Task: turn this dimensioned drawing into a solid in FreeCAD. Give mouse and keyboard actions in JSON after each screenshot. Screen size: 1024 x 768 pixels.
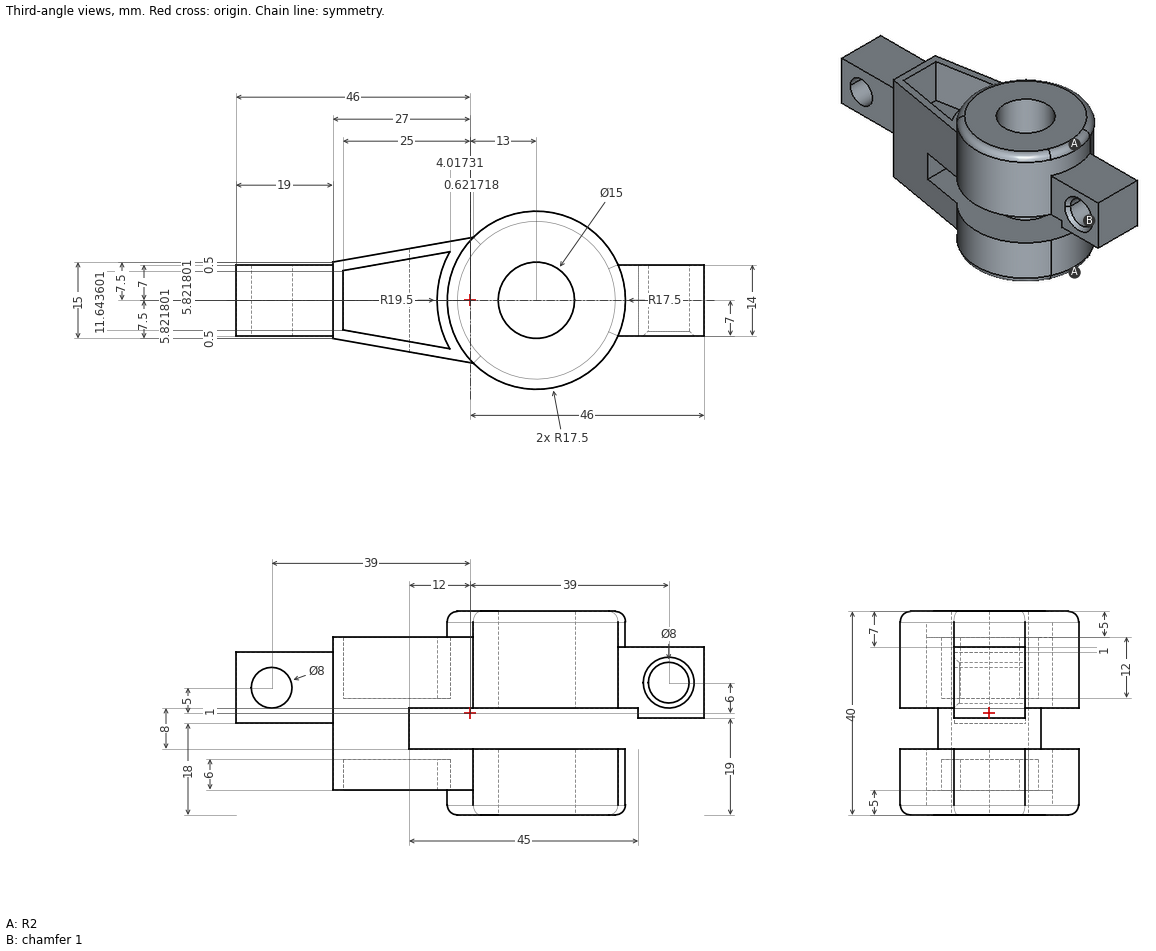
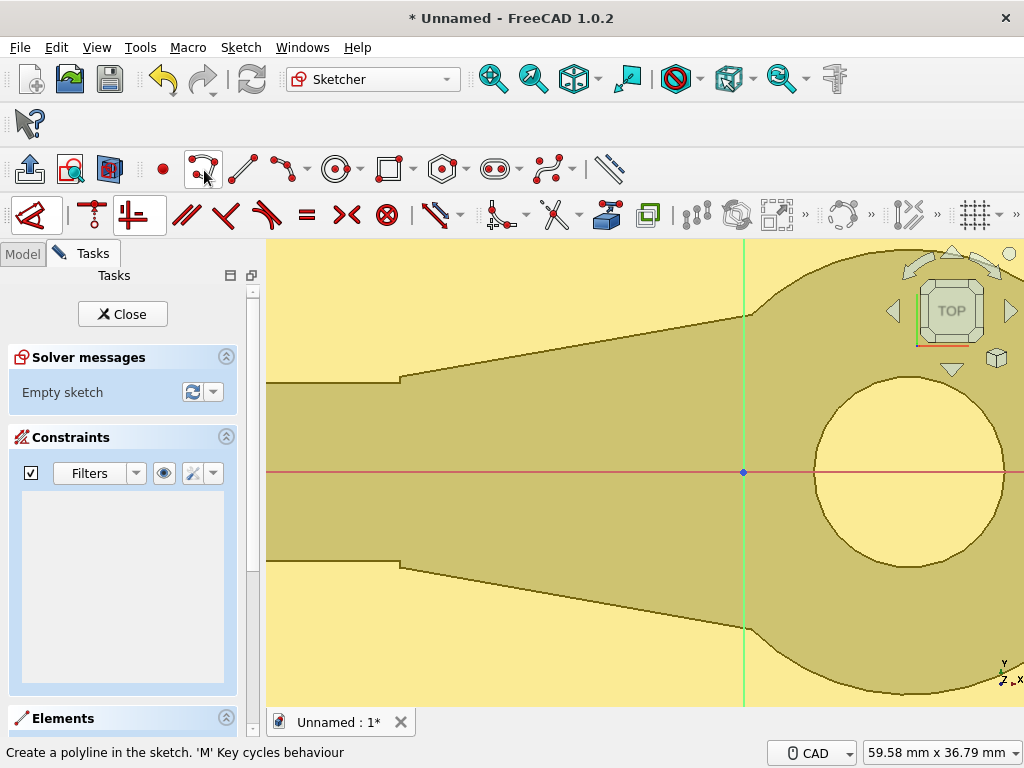
{"action": "scroll", "coordinate": [752, 630], "scroll_direction": "up", "scroll_amount": 4}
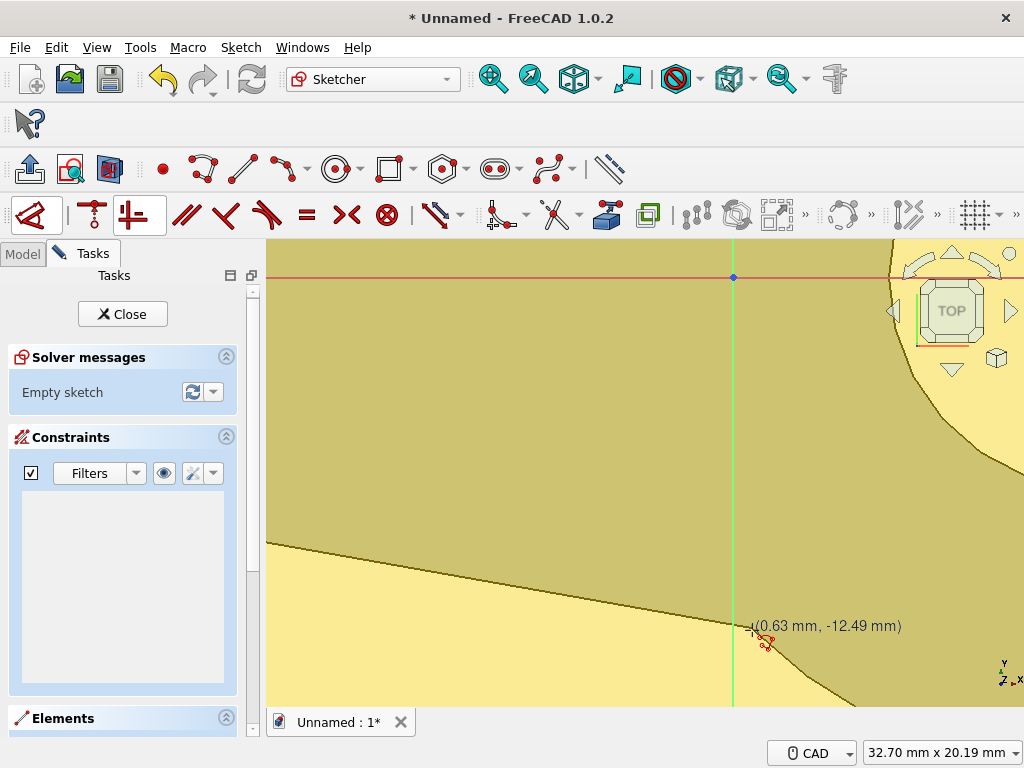
{"action": "left_click", "coordinate": [751, 628]}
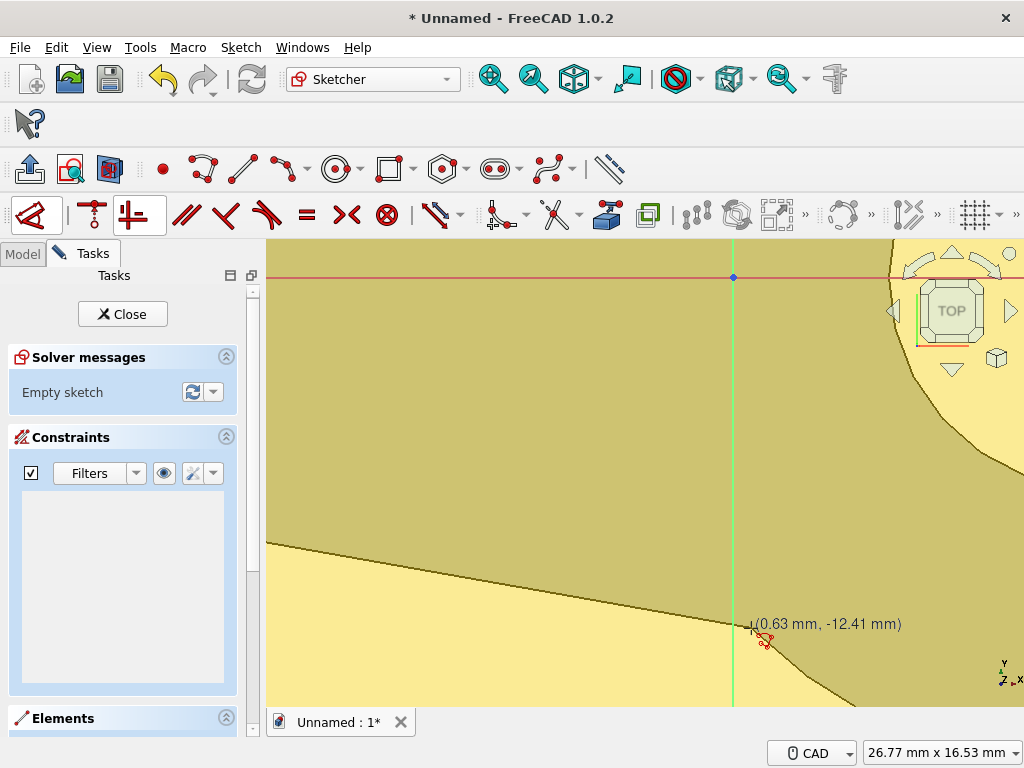
{"action": "scroll", "coordinate": [753, 632], "scroll_direction": "down", "scroll_amount": 4}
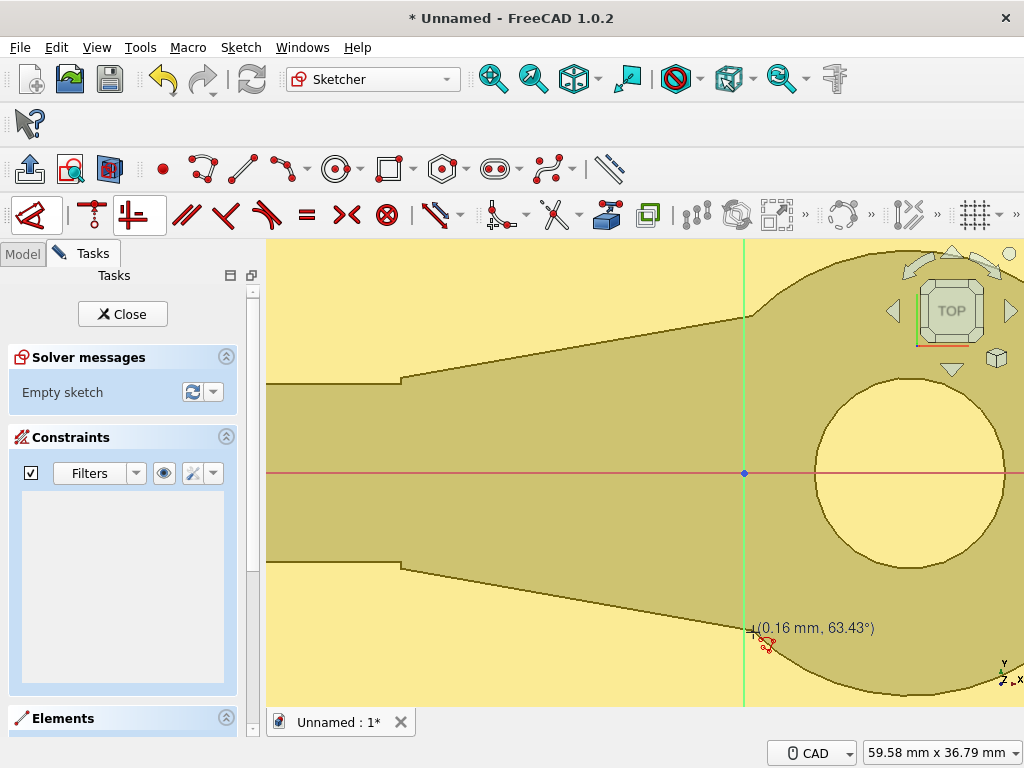
{"action": "left_click", "coordinate": [401, 569]}
{"action": "left_click", "coordinate": [401, 378]}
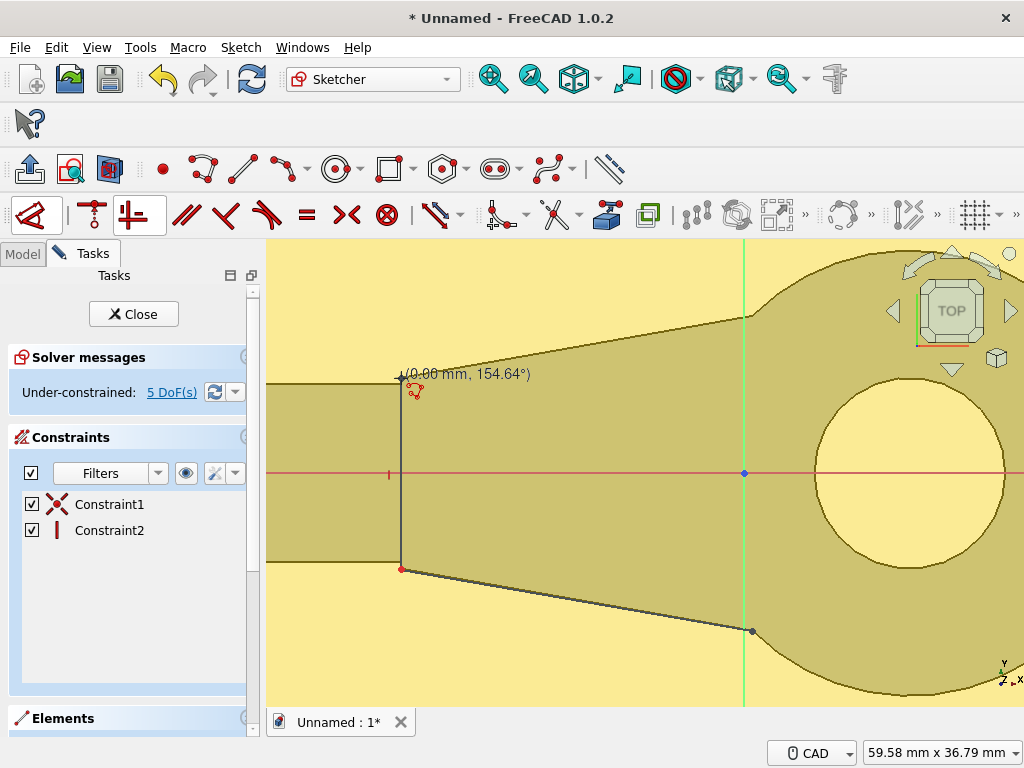
{"action": "scroll", "coordinate": [752, 316], "scroll_direction": "up", "scroll_amount": 4}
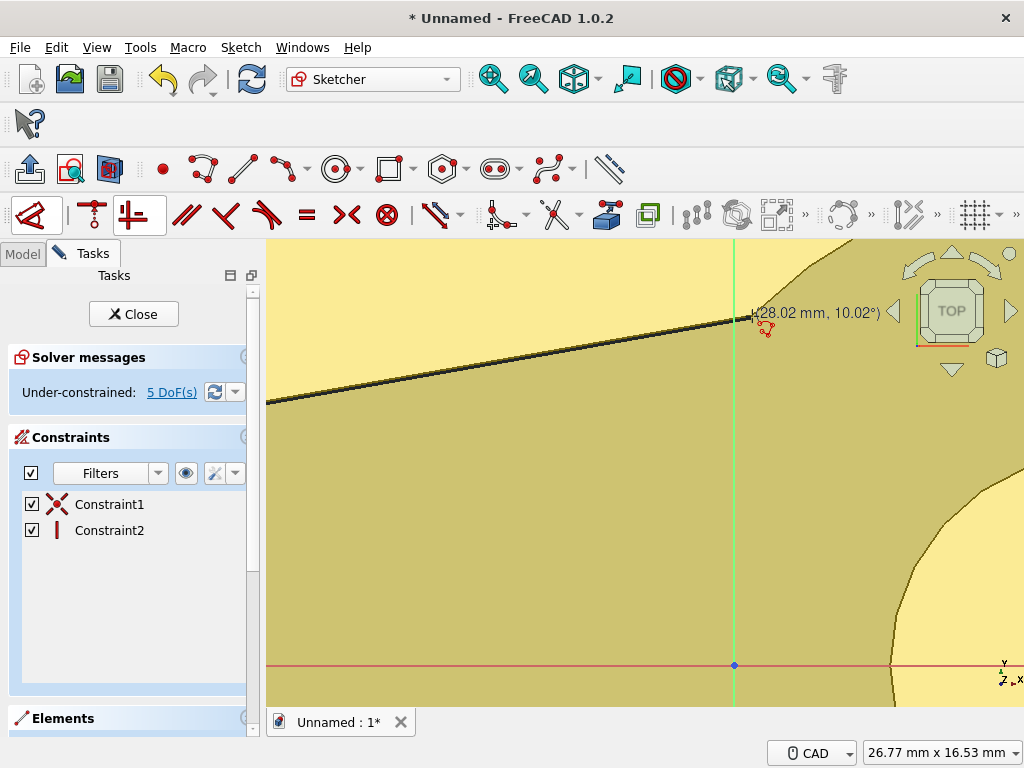
{"action": "left_click", "coordinate": [752, 316]}
{"action": "right_click", "coordinate": [752, 316]}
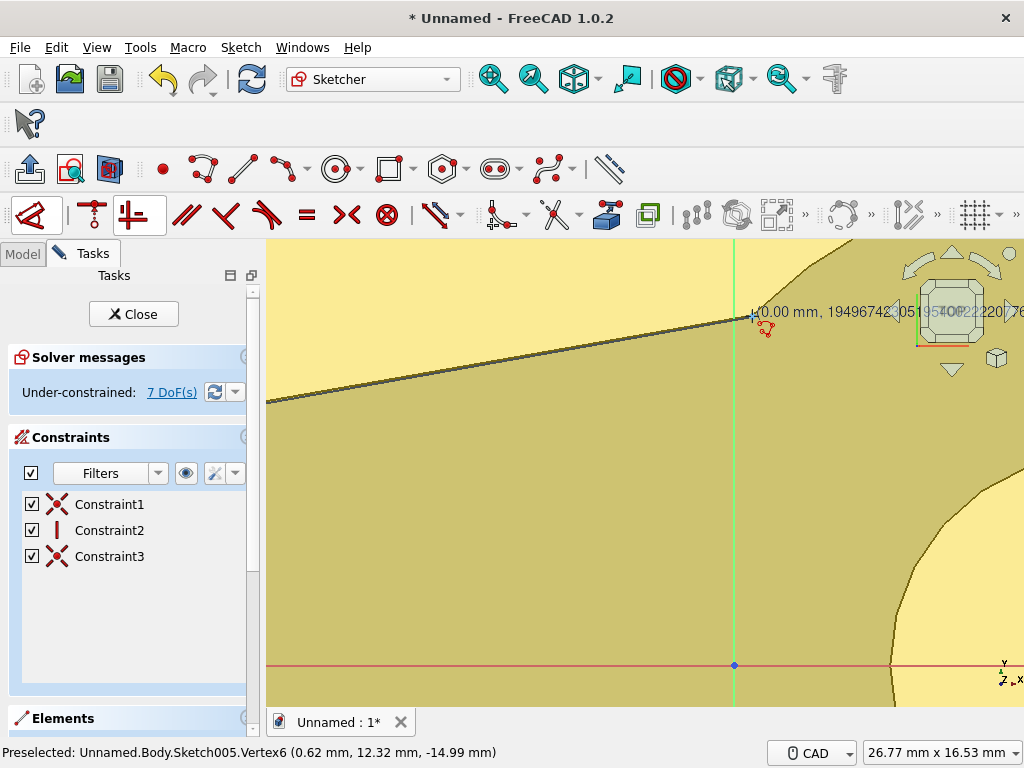
{"action": "left_click", "coordinate": [284, 170]}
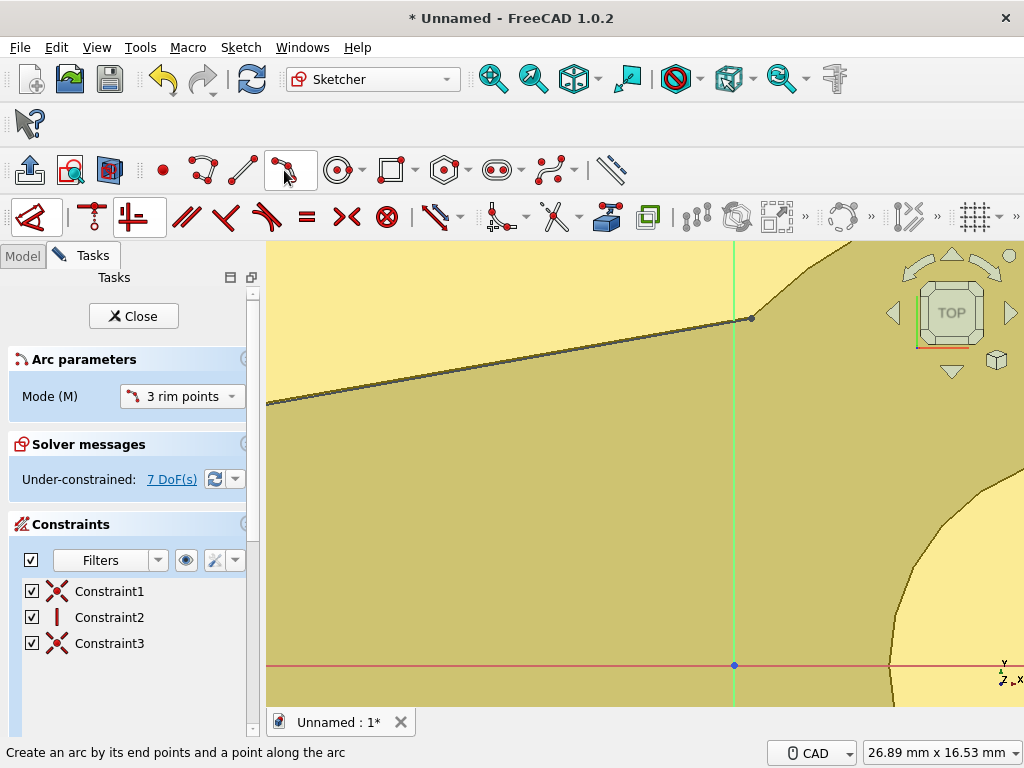
{"action": "left_click", "coordinate": [752, 319]}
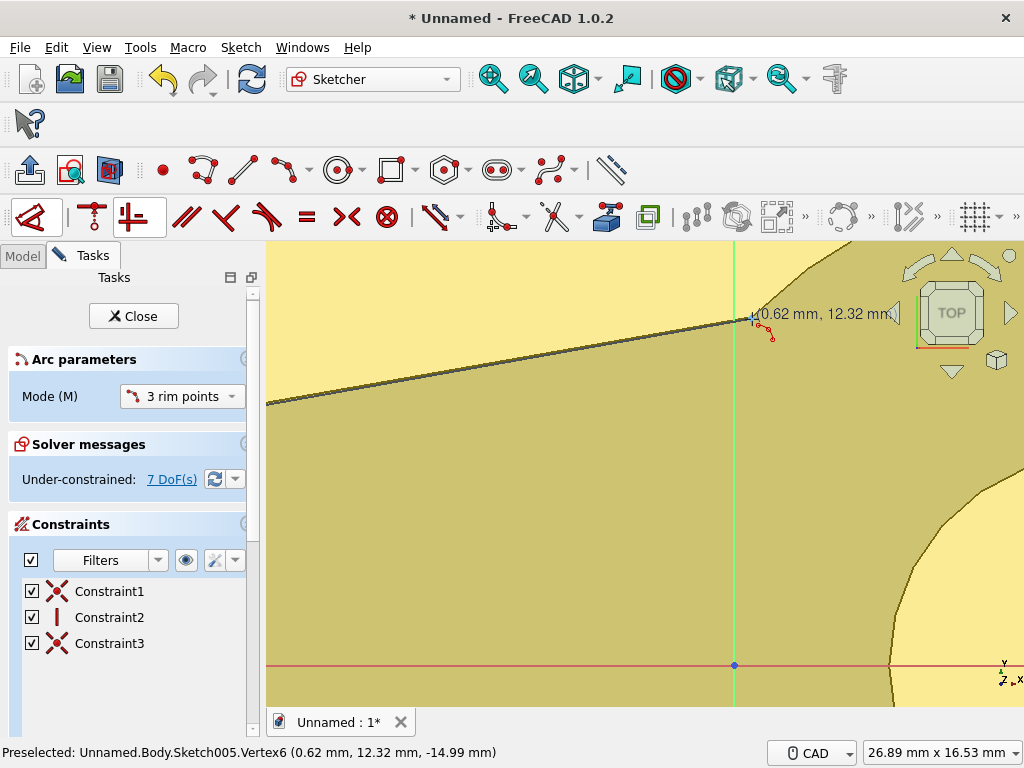
{"action": "scroll", "coordinate": [751, 317], "scroll_direction": "down", "scroll_amount": 4}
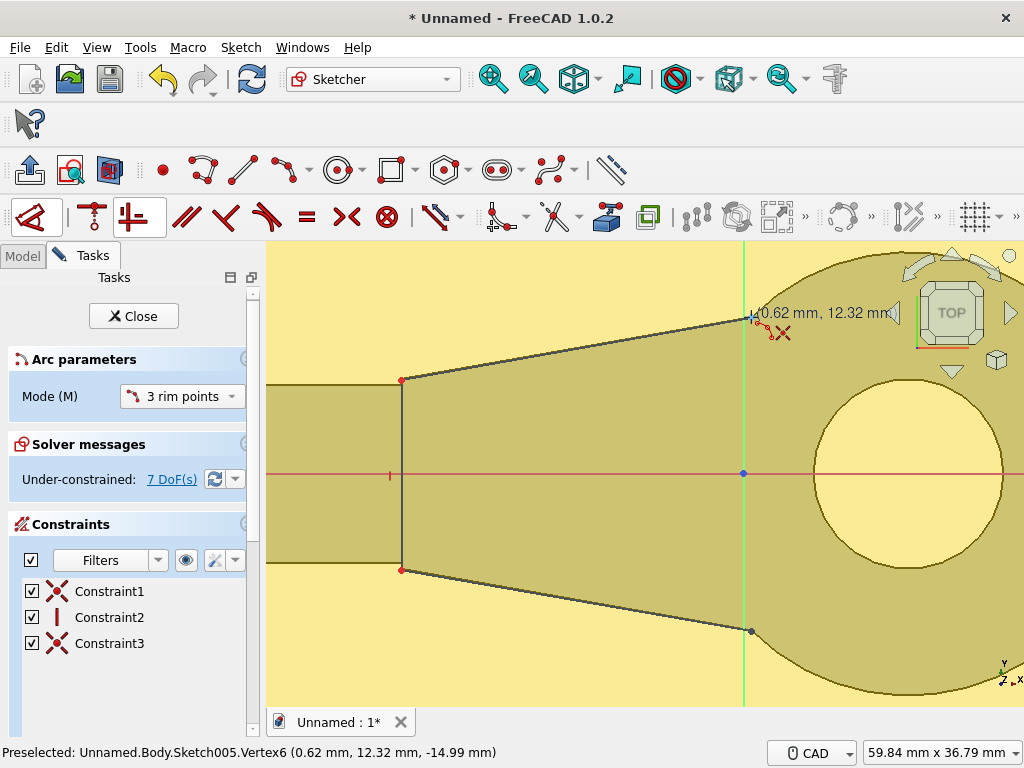
{"action": "scroll", "coordinate": [752, 631], "scroll_direction": "up", "scroll_amount": 4}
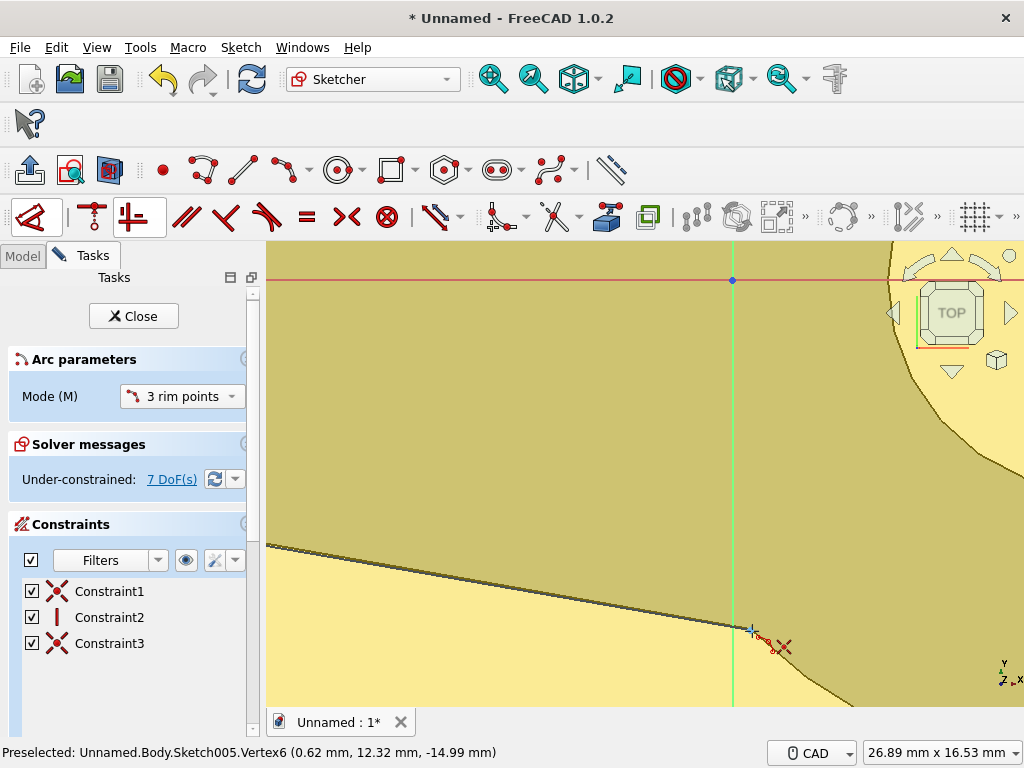
{"action": "left_click", "coordinate": [751, 630]}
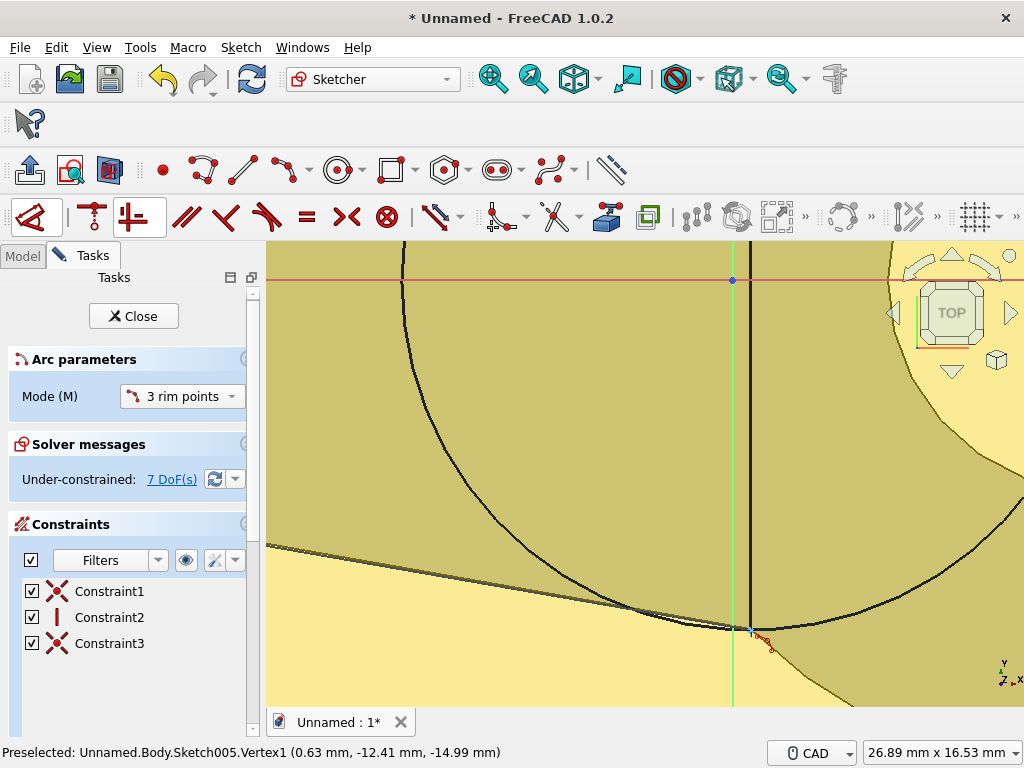
{"action": "scroll", "coordinate": [752, 632], "scroll_direction": "down", "scroll_amount": 4}